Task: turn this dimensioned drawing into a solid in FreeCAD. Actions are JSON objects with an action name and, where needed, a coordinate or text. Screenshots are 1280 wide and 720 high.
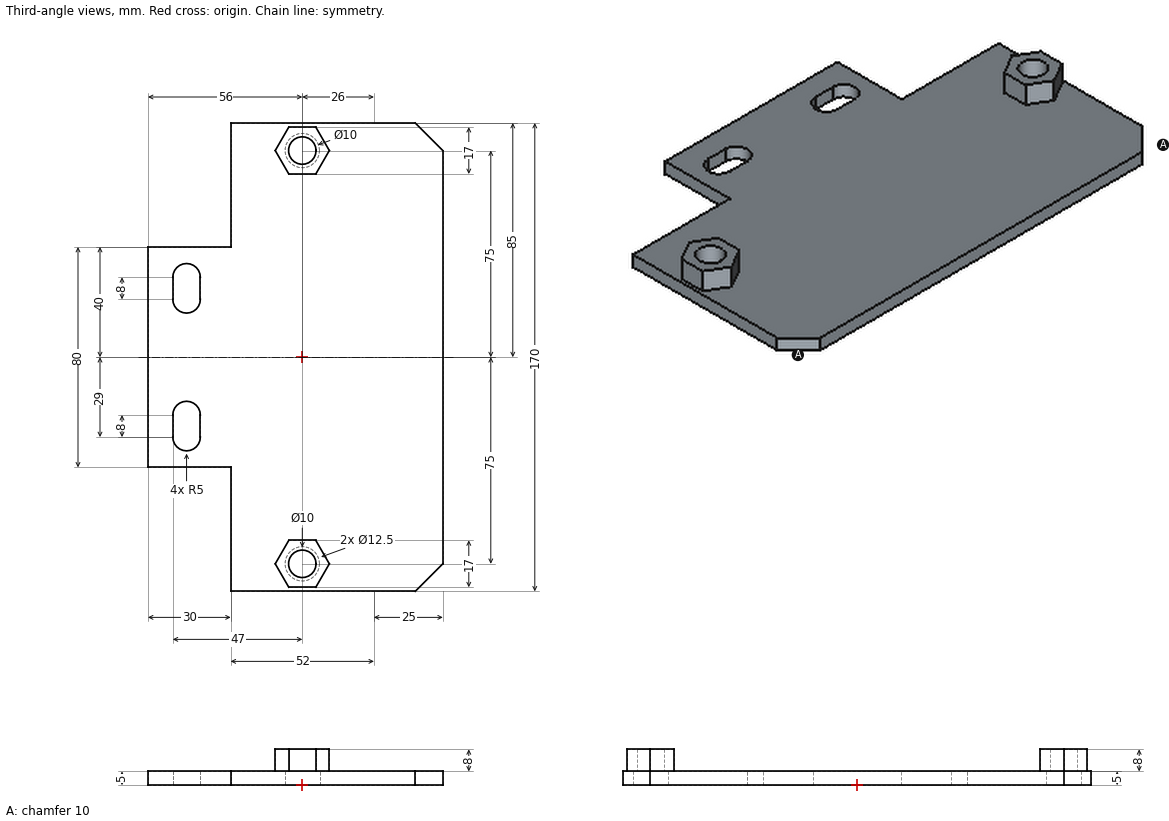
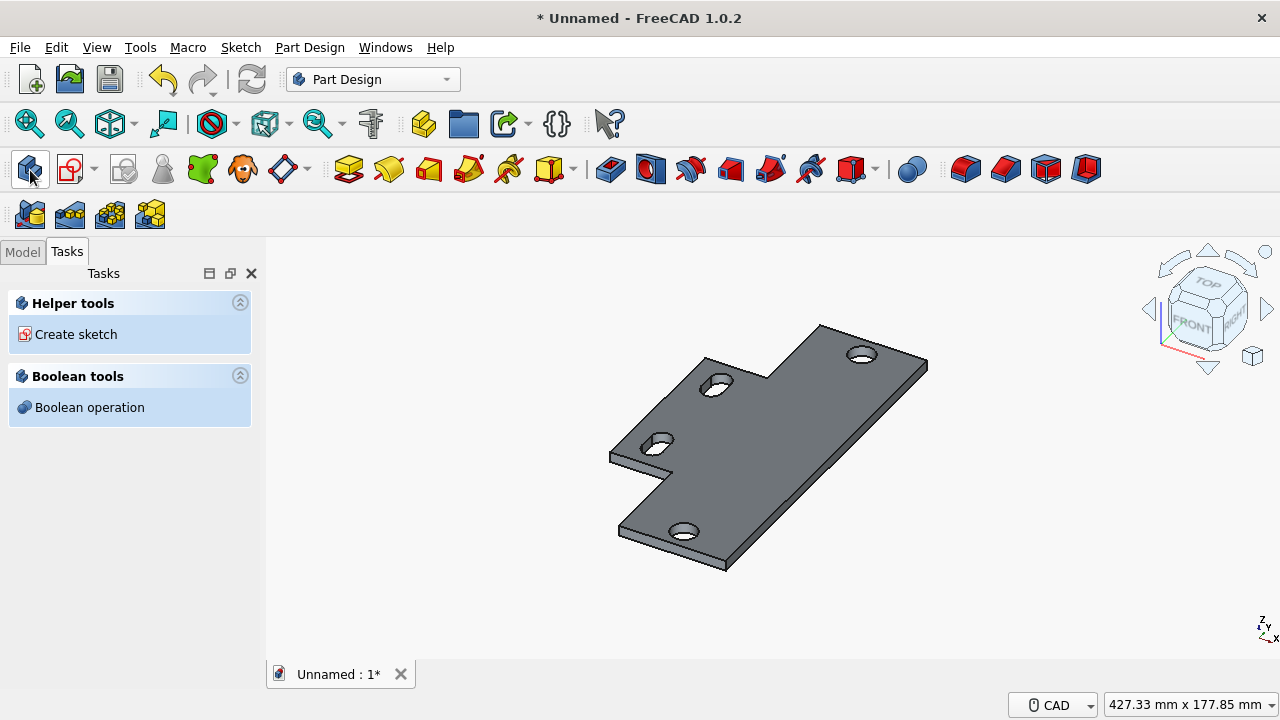
{"action": "left_click", "coordinate": [23, 251]}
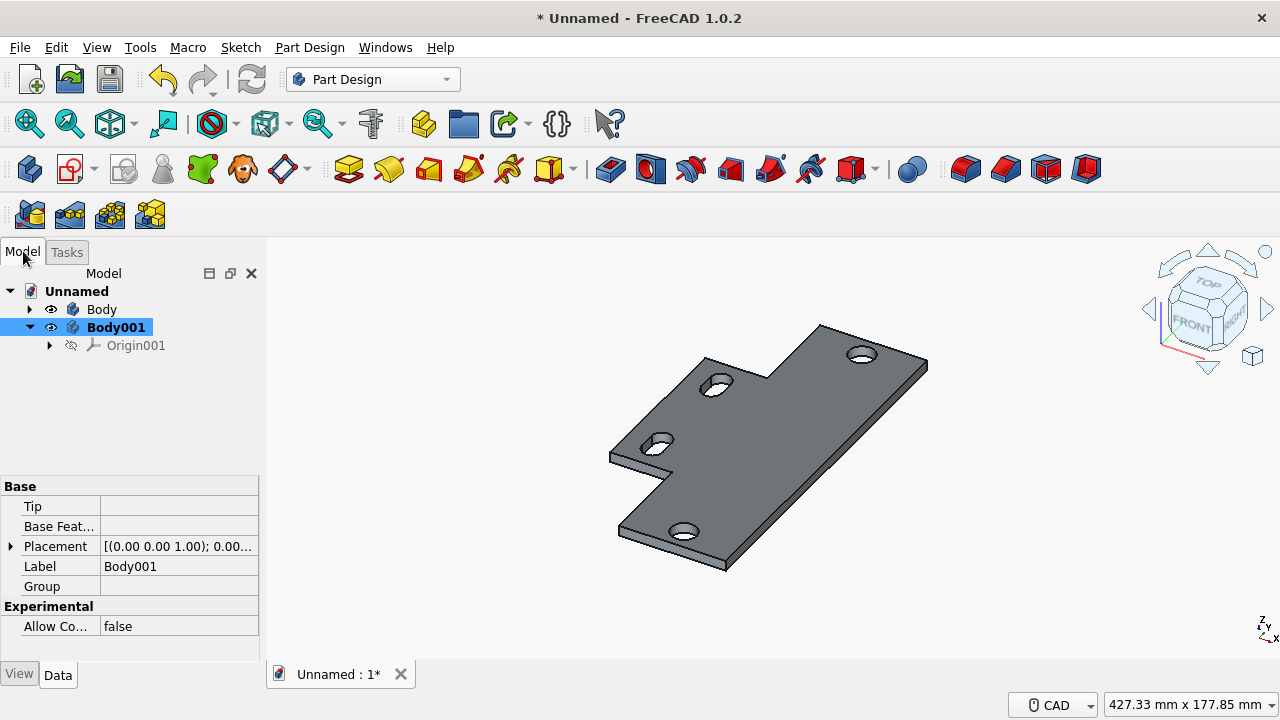
{"action": "left_click", "coordinate": [50, 345]}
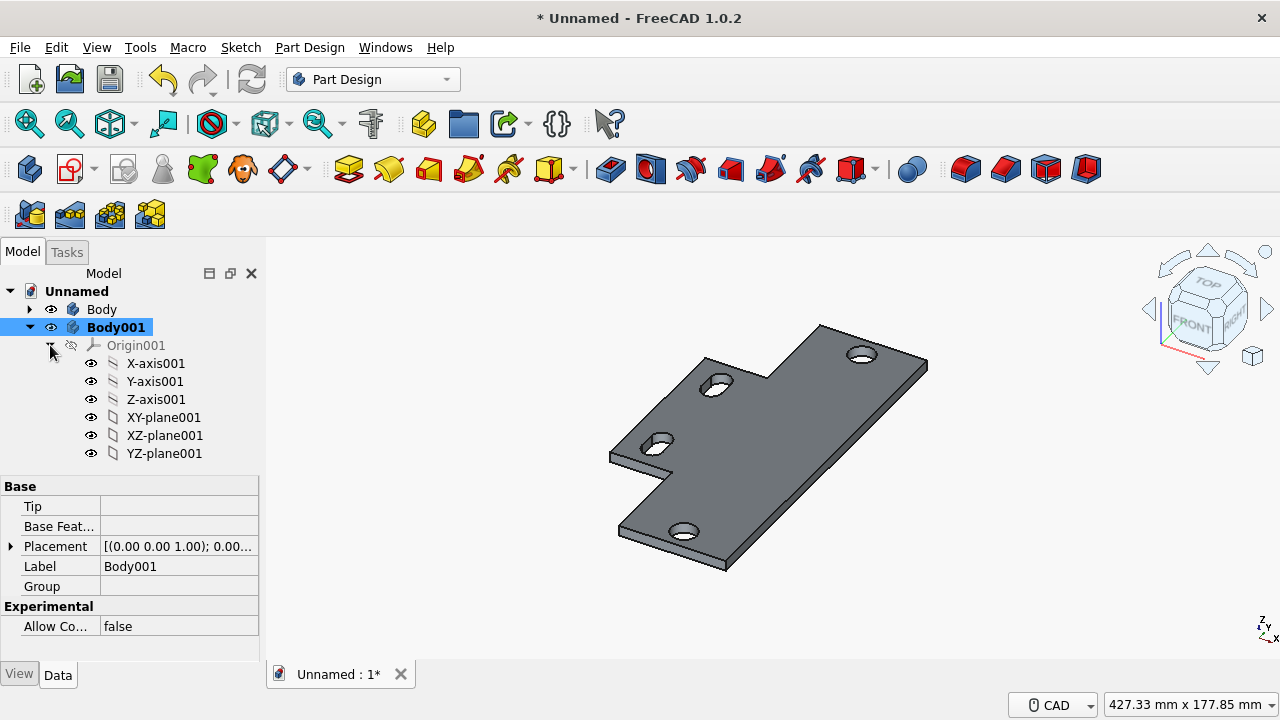
{"action": "left_click", "coordinate": [136, 417]}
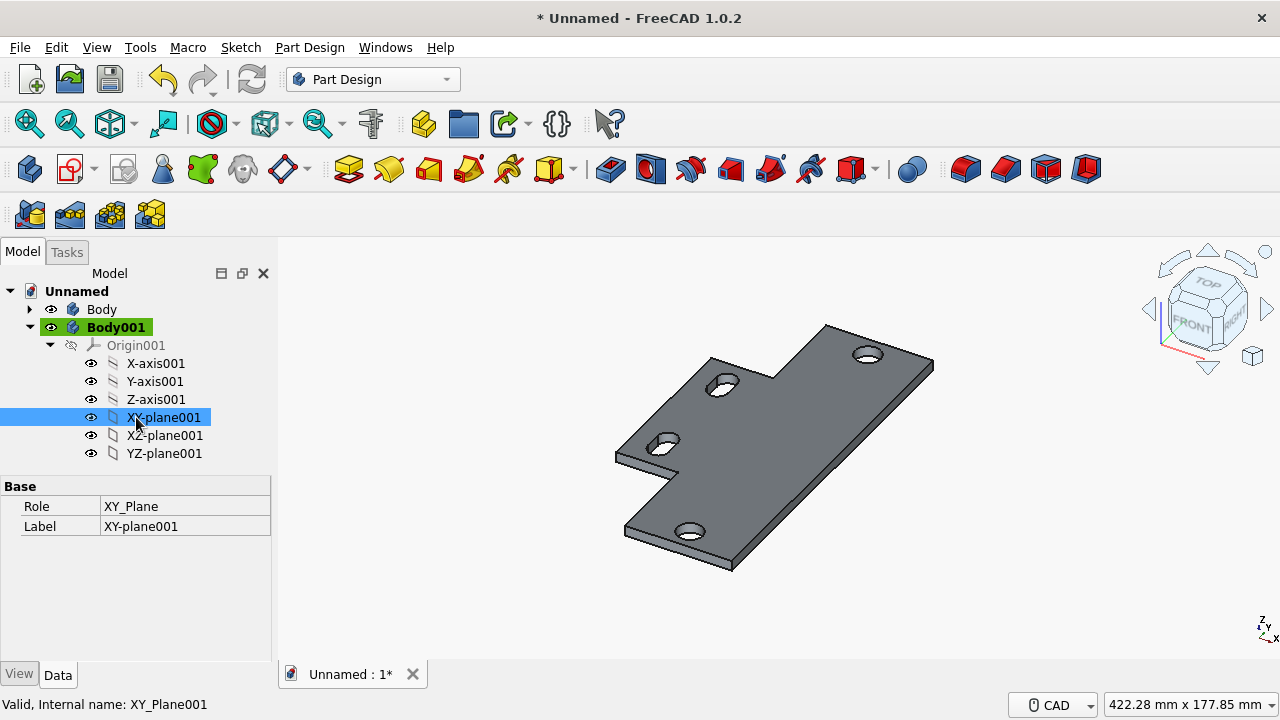
{"action": "left_click", "coordinate": [284, 170]}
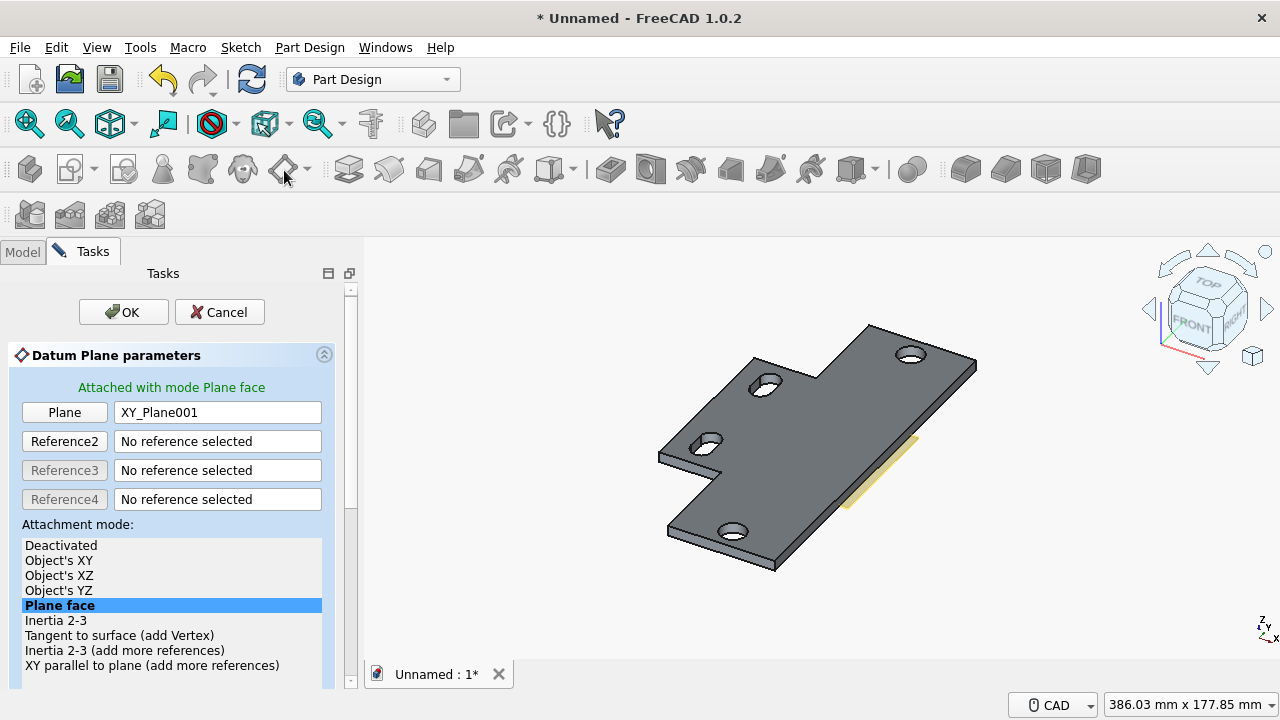
{"action": "scroll", "coordinate": [351, 486], "scroll_direction": "down", "scroll_amount": 4}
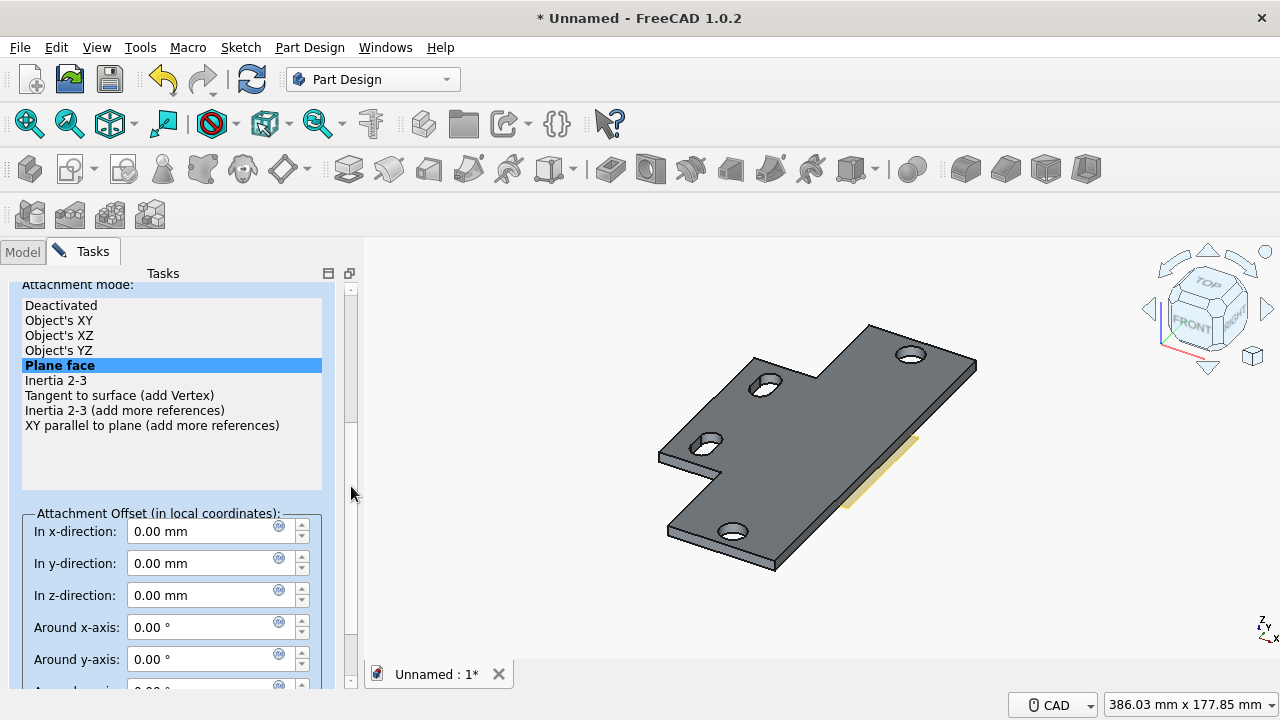
{"action": "triple_click", "coordinate": [210, 595]}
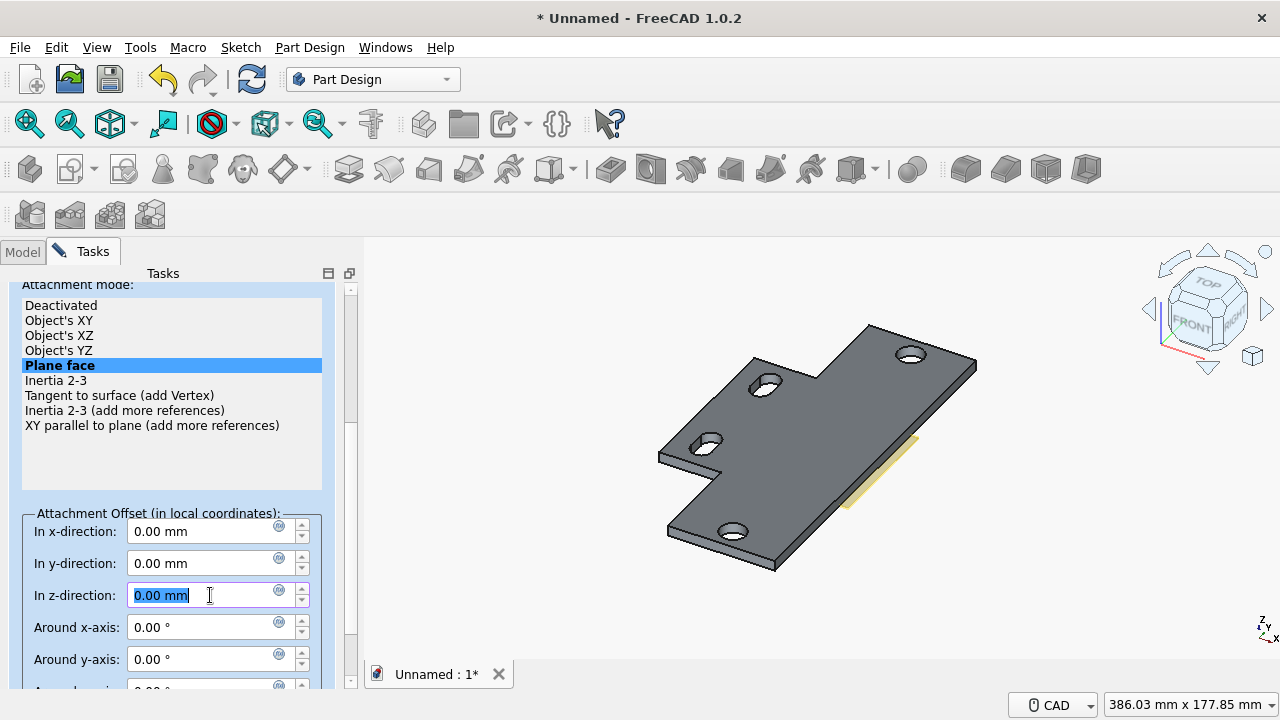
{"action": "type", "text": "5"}
{"action": "key", "text": "Tab"}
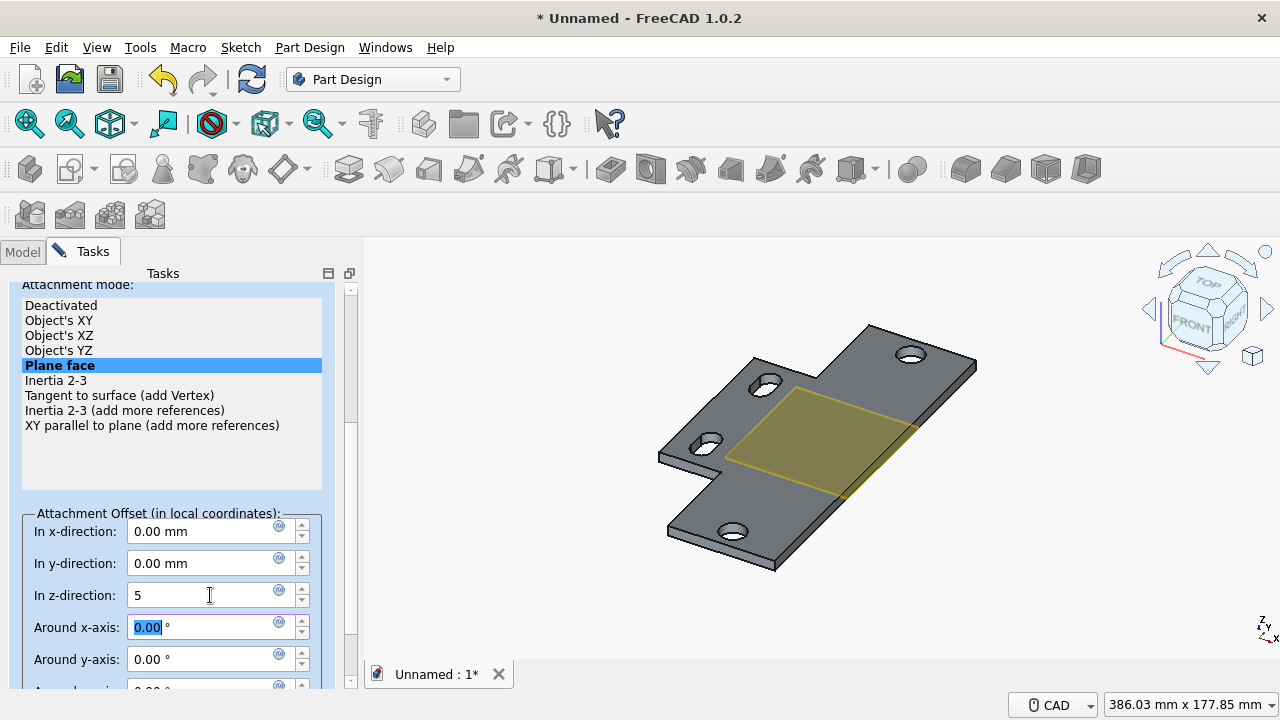
{"action": "scroll", "coordinate": [351, 486], "scroll_direction": "up", "scroll_amount": 5}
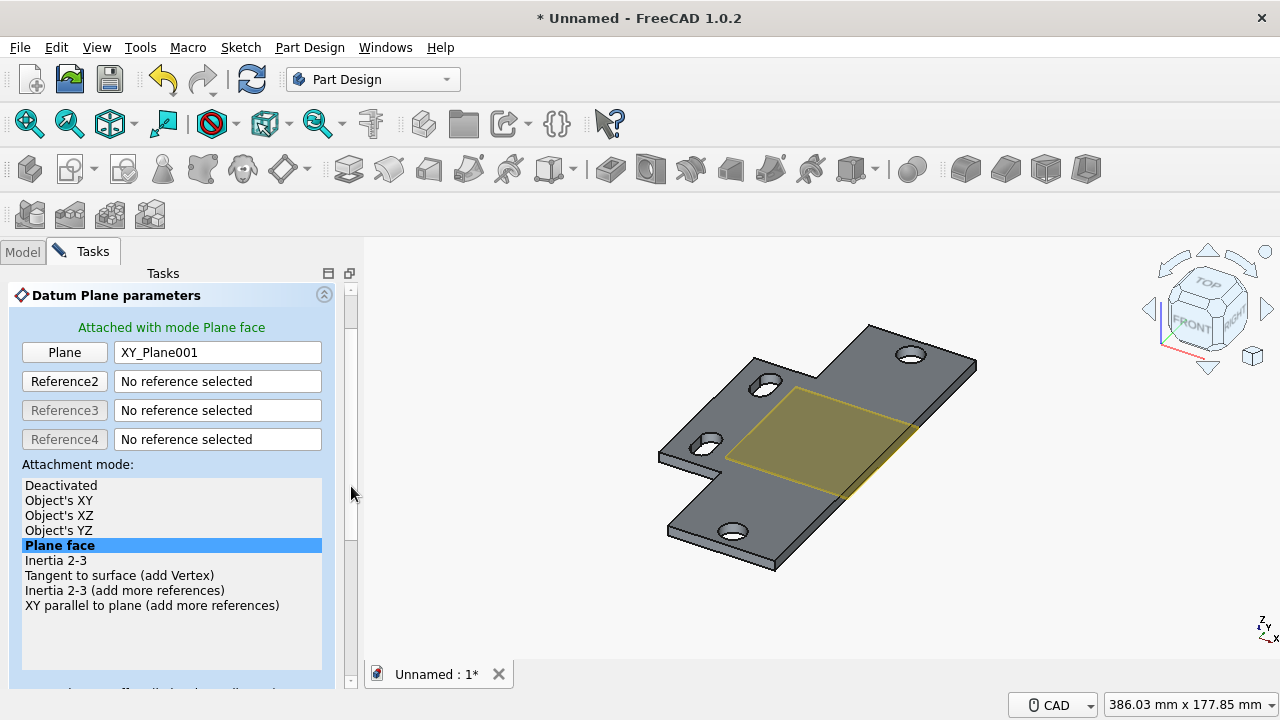
{"action": "left_click", "coordinate": [124, 312]}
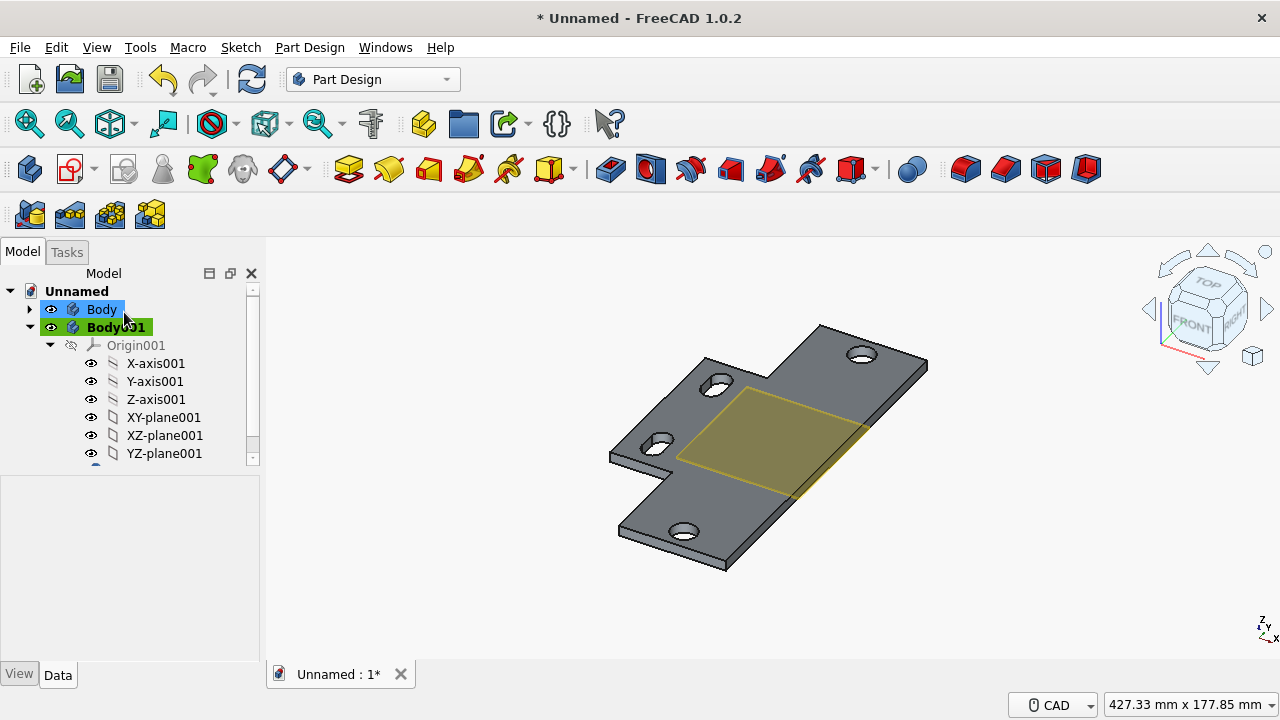
{"action": "scroll", "coordinate": [100, 377], "scroll_direction": "down", "scroll_amount": 3}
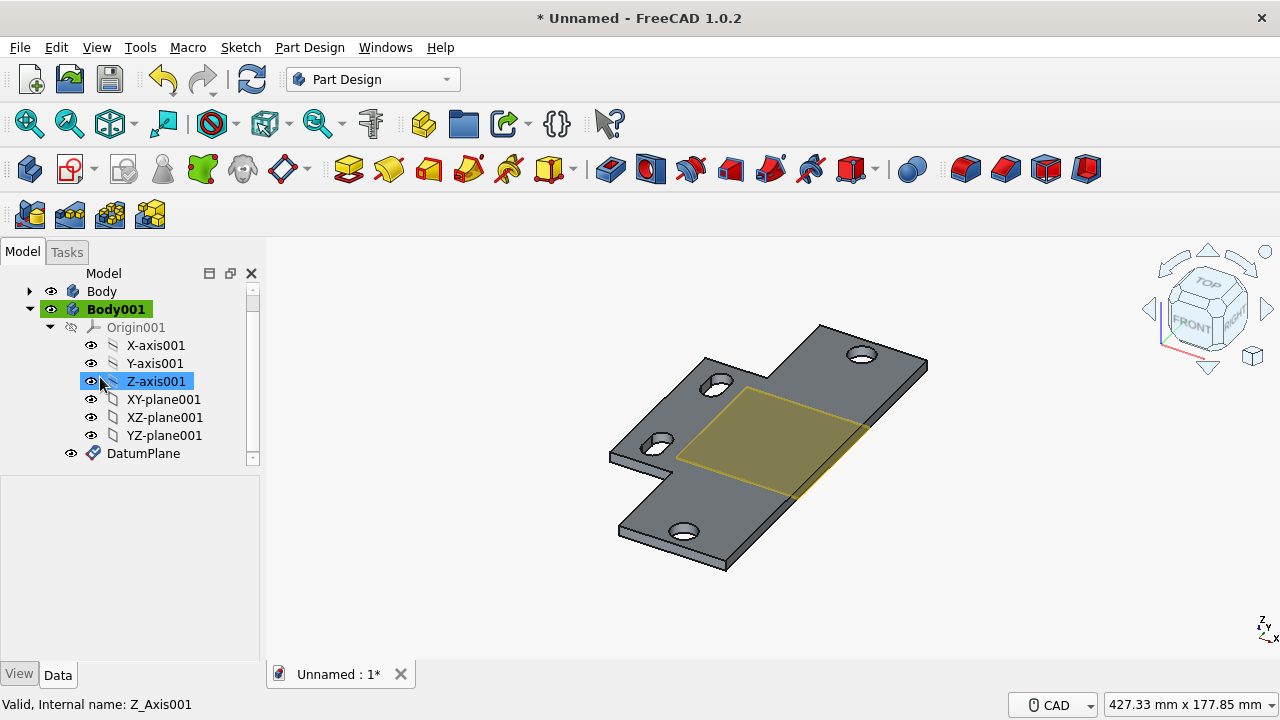
{"action": "left_click", "coordinate": [116, 453]}